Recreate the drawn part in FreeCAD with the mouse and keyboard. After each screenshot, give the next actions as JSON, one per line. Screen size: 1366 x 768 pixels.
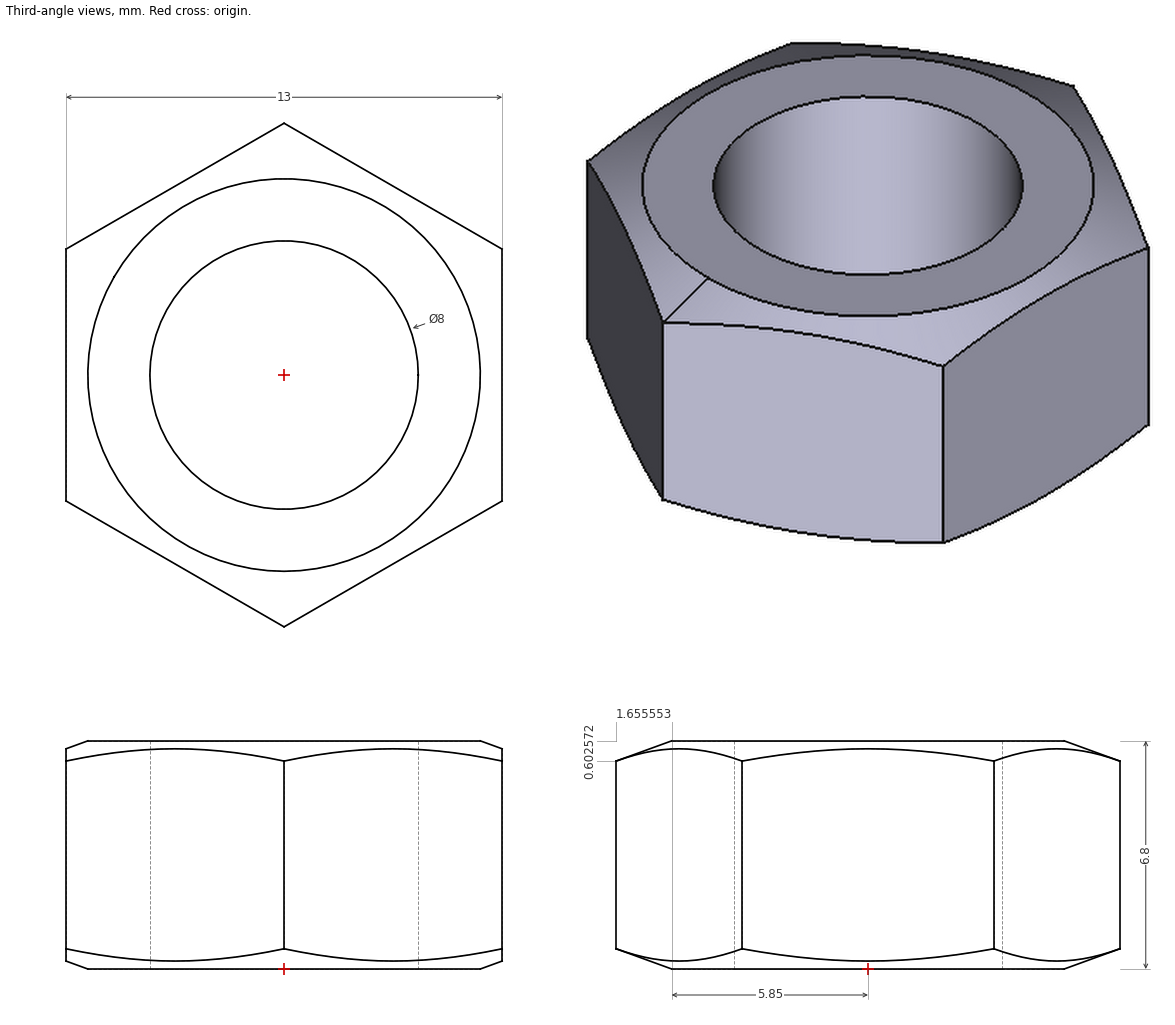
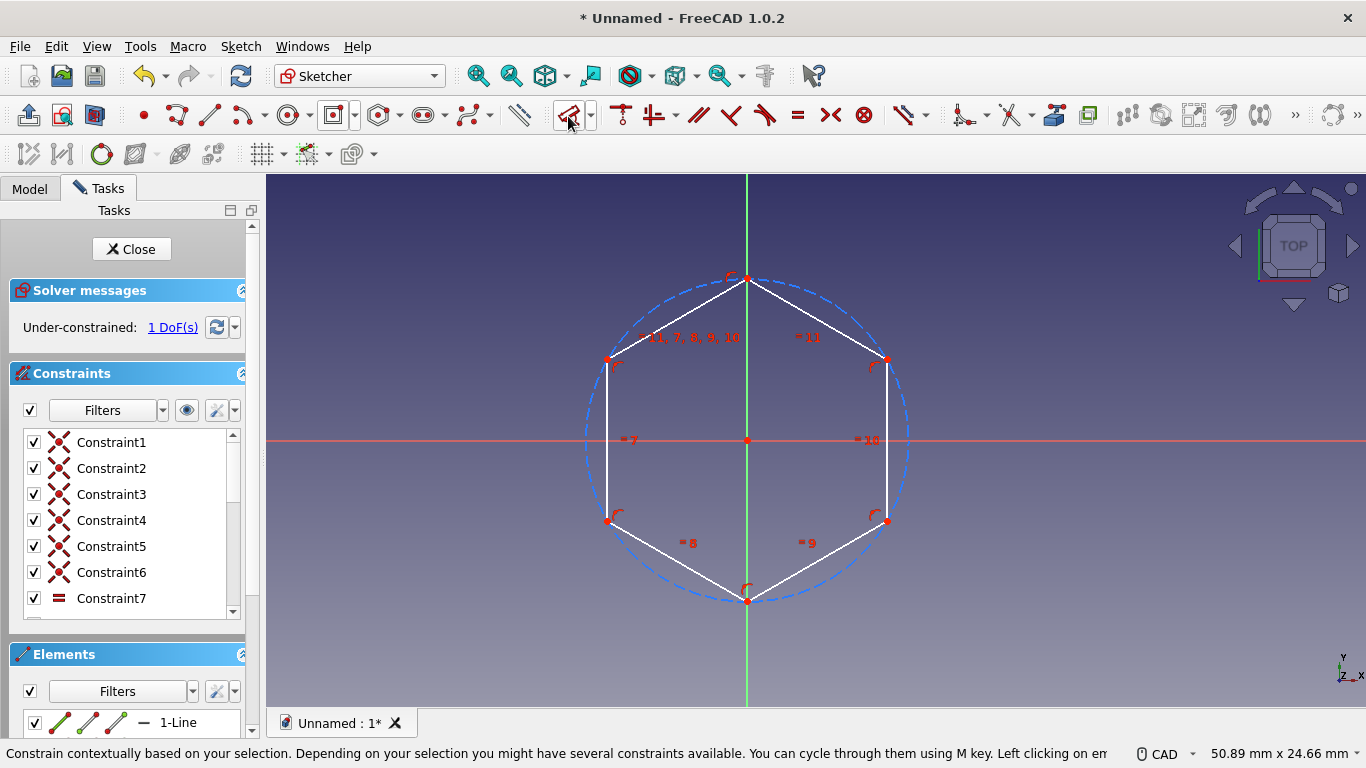
{"action": "left_click", "coordinate": [607, 360]}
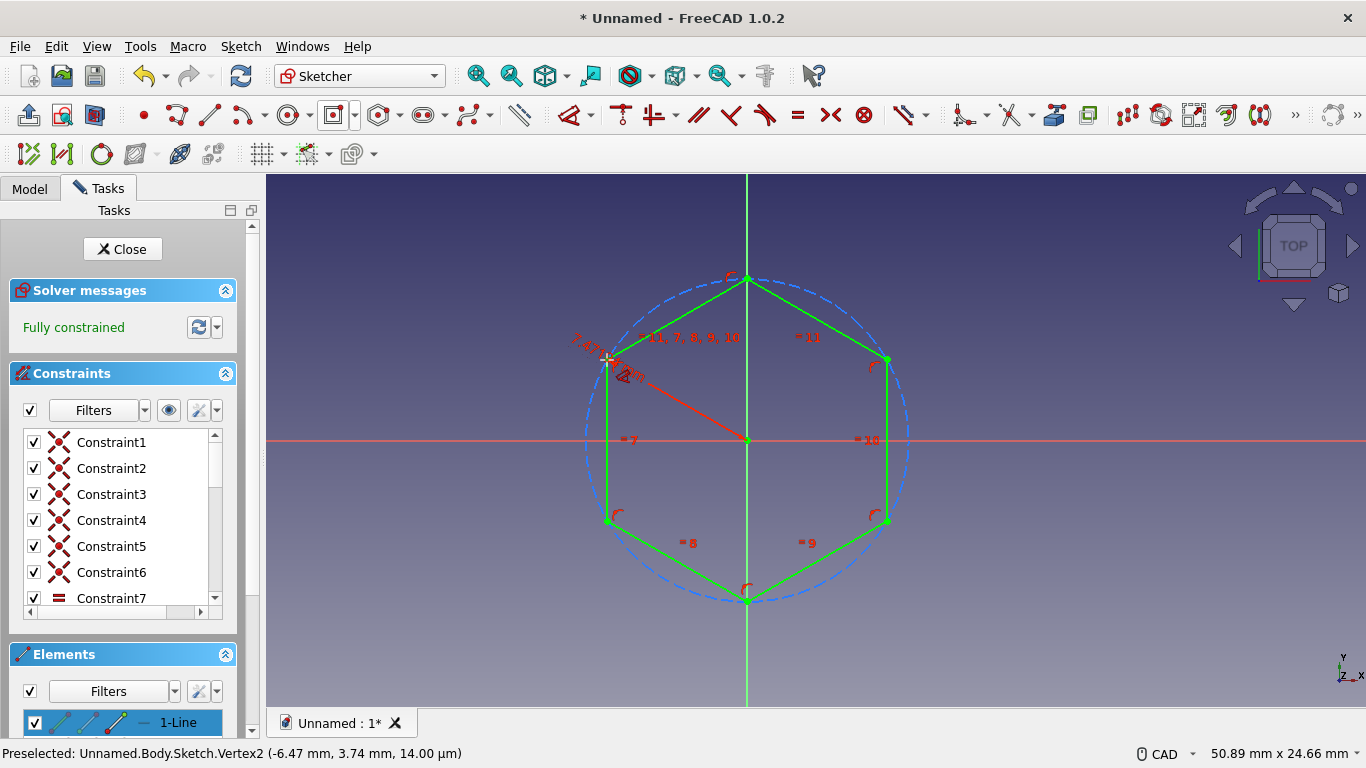
{"action": "left_click", "coordinate": [887, 521]}
{"action": "left_click", "coordinate": [683, 603]}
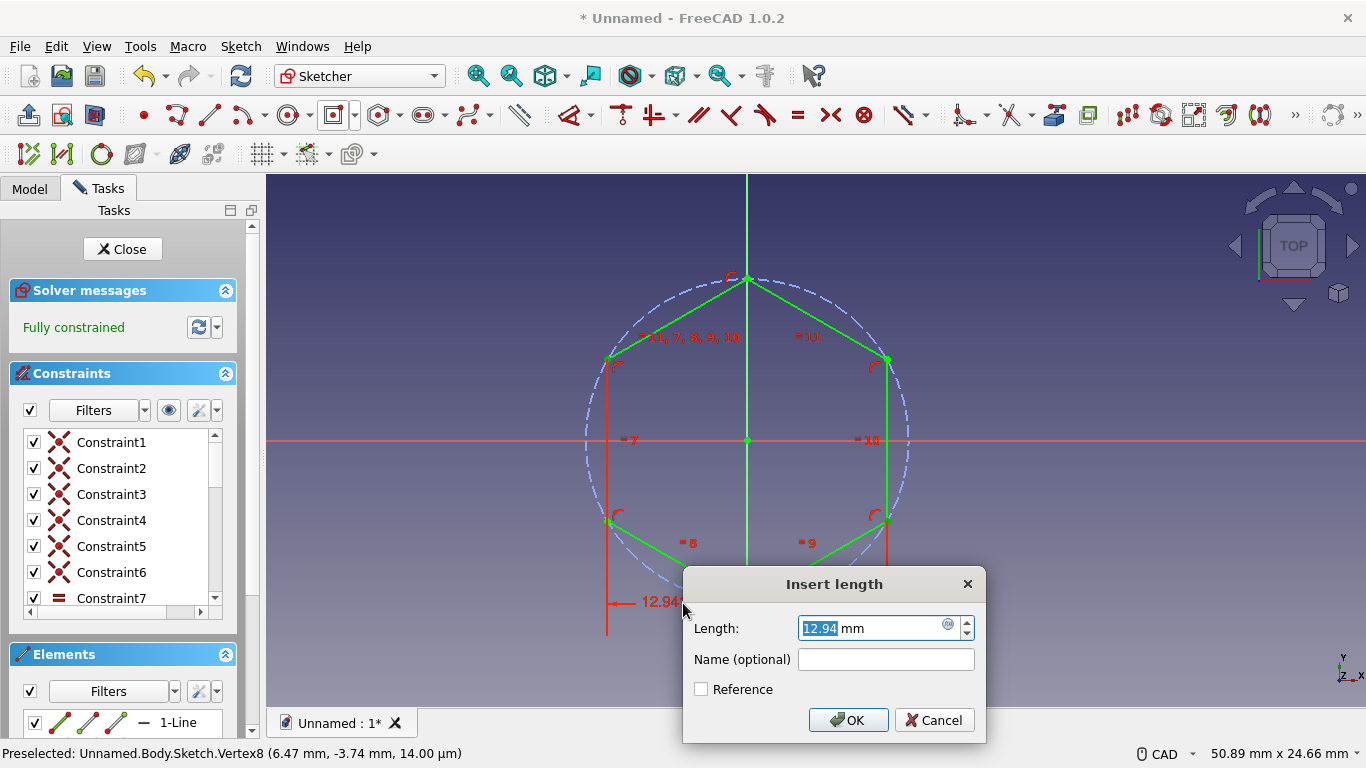
{"action": "type", "text": "13"}
{"action": "key", "text": "Return"}
{"action": "key", "text": "Escape"}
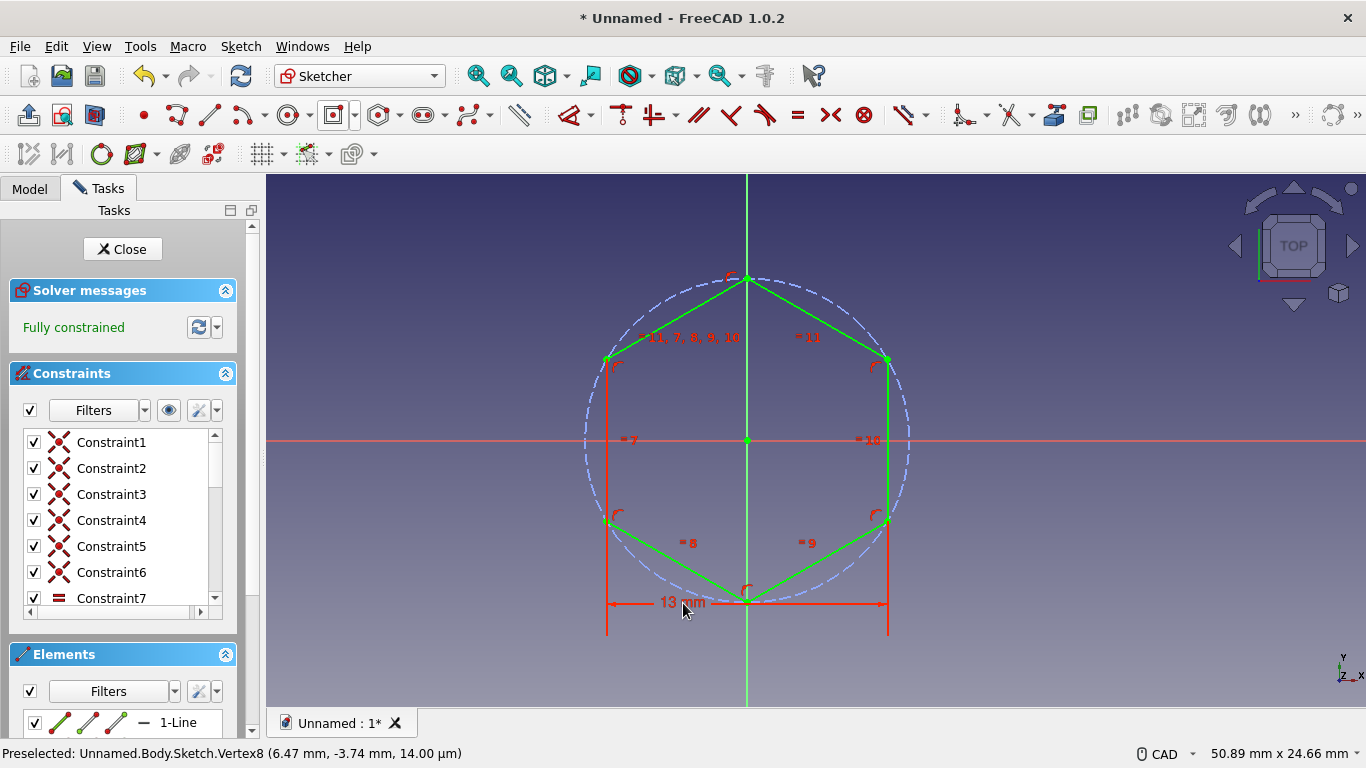
{"action": "left_click", "coordinate": [123, 249]}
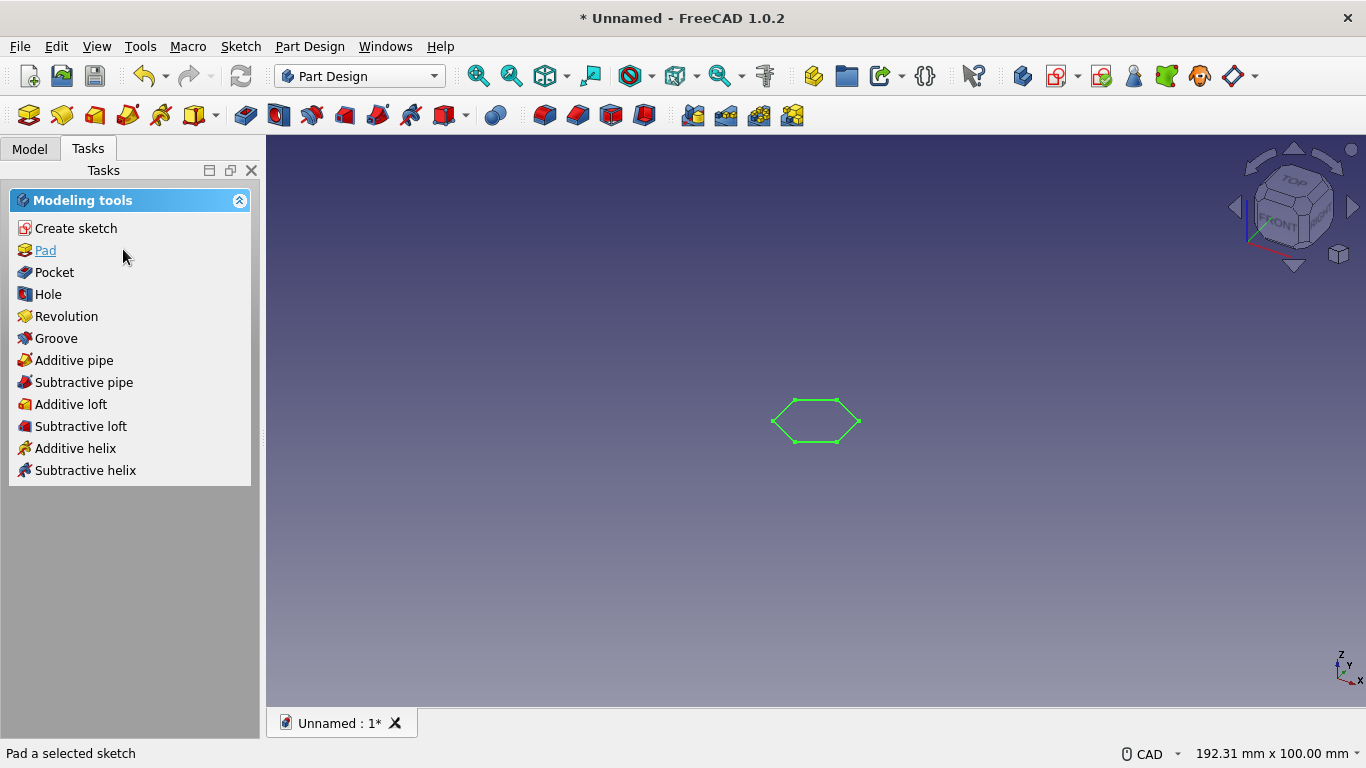
{"action": "left_click", "coordinate": [29, 116]}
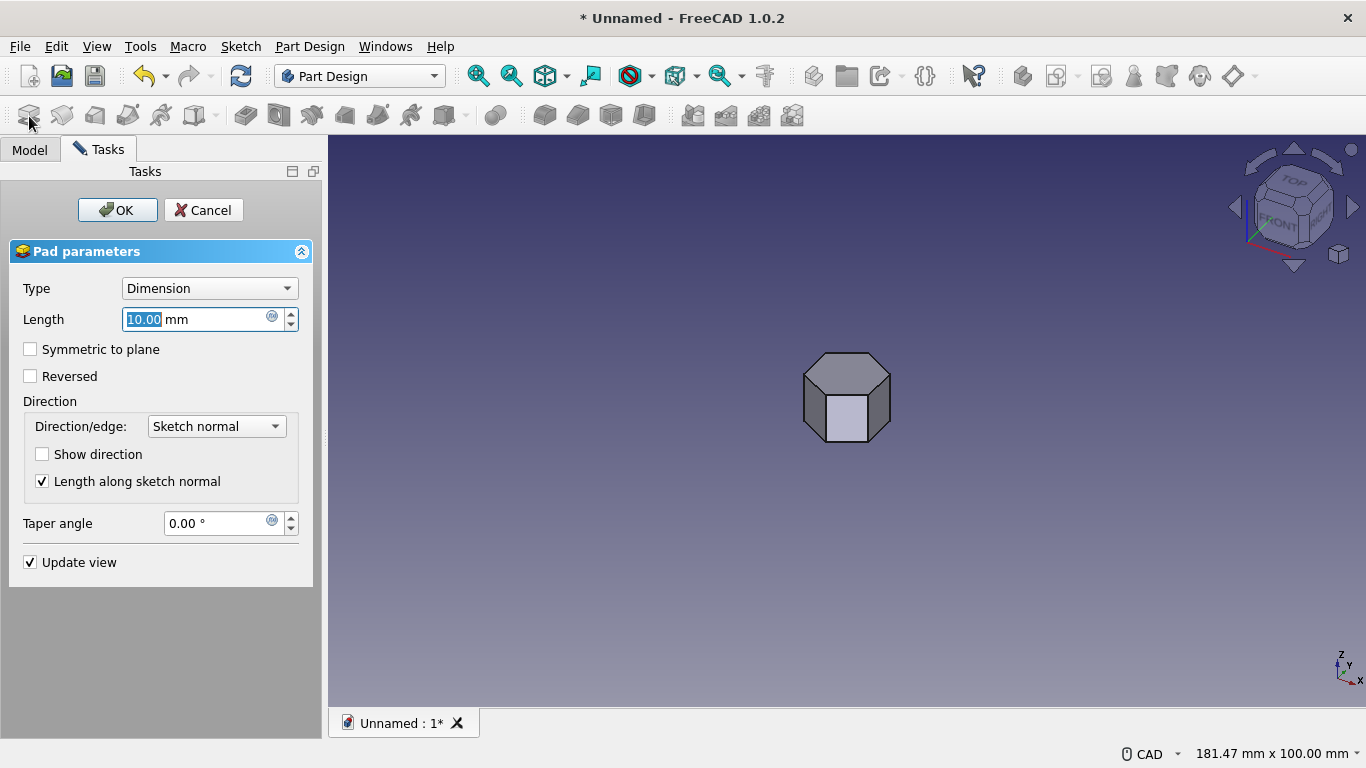
{"action": "type", "text": "6.8"}
{"action": "key", "text": "Tab"}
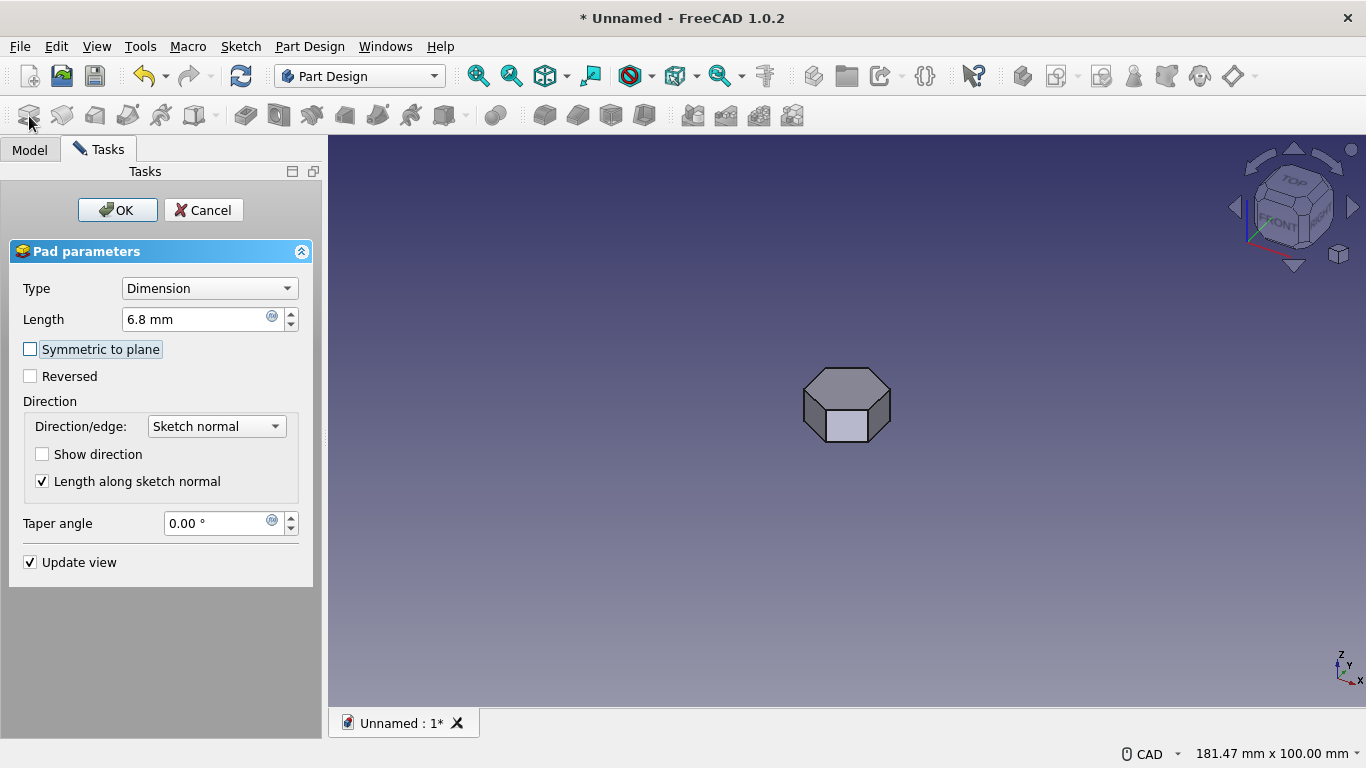
{"action": "left_click", "coordinate": [118, 210]}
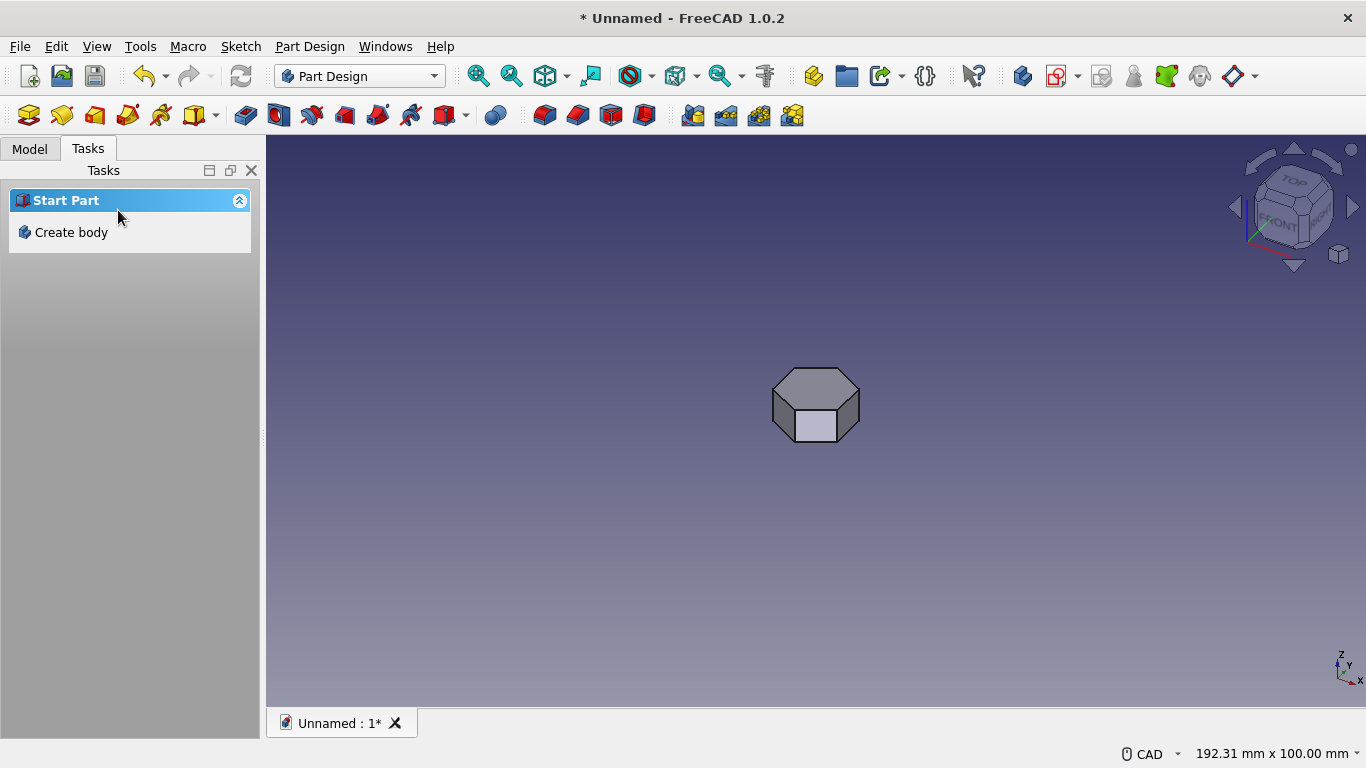
{"action": "left_click", "coordinate": [479, 76]}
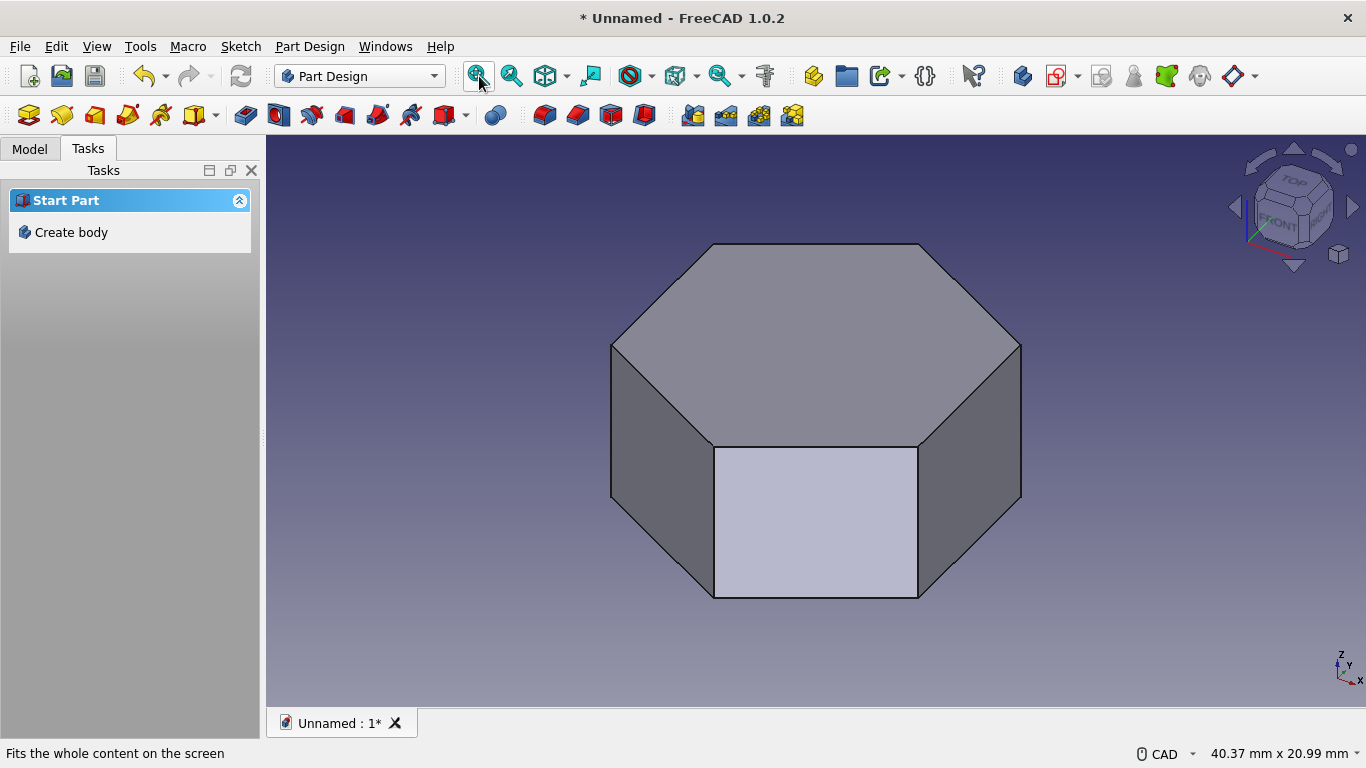
{"action": "left_click", "coordinate": [1056, 76]}